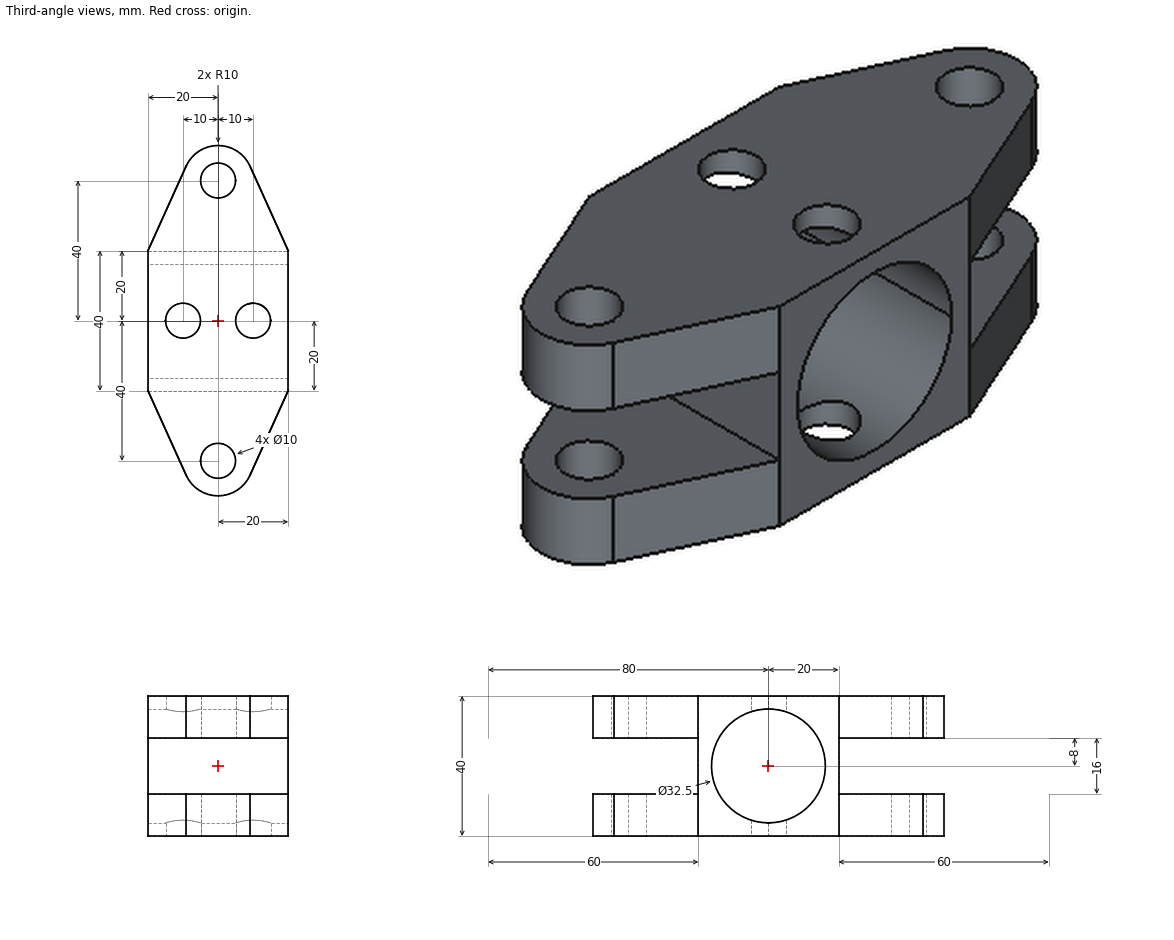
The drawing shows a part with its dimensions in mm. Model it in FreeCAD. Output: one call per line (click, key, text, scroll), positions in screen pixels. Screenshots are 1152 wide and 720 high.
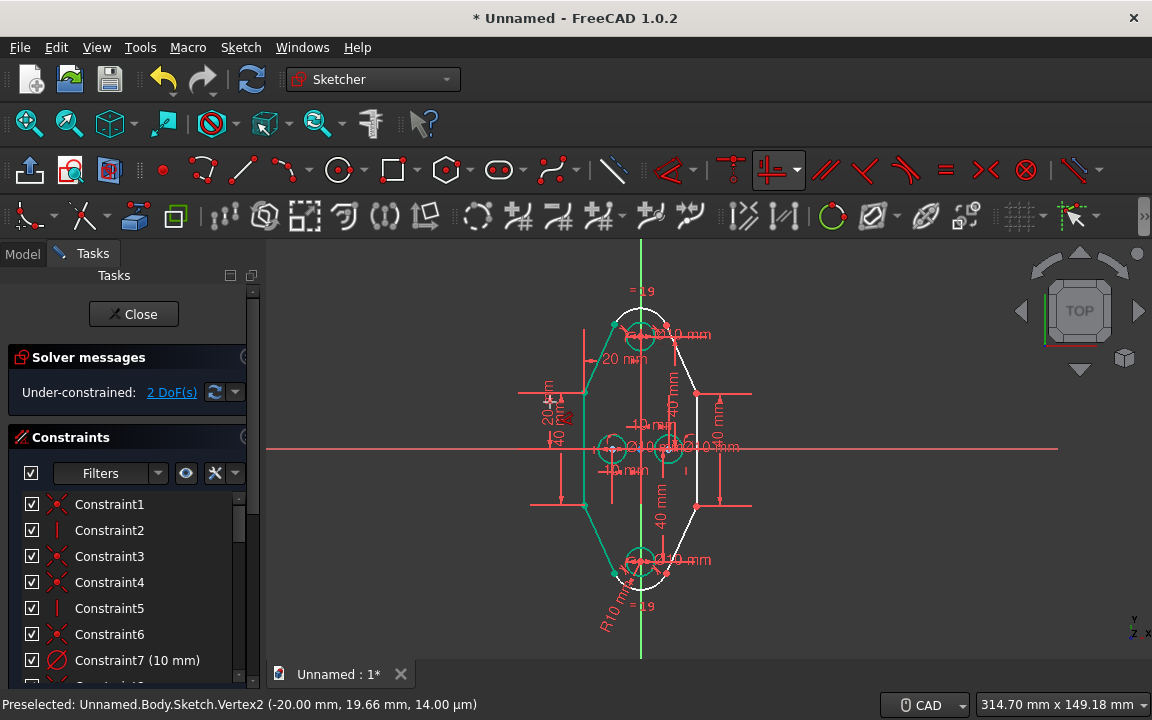
click(697, 506)
click(689, 564)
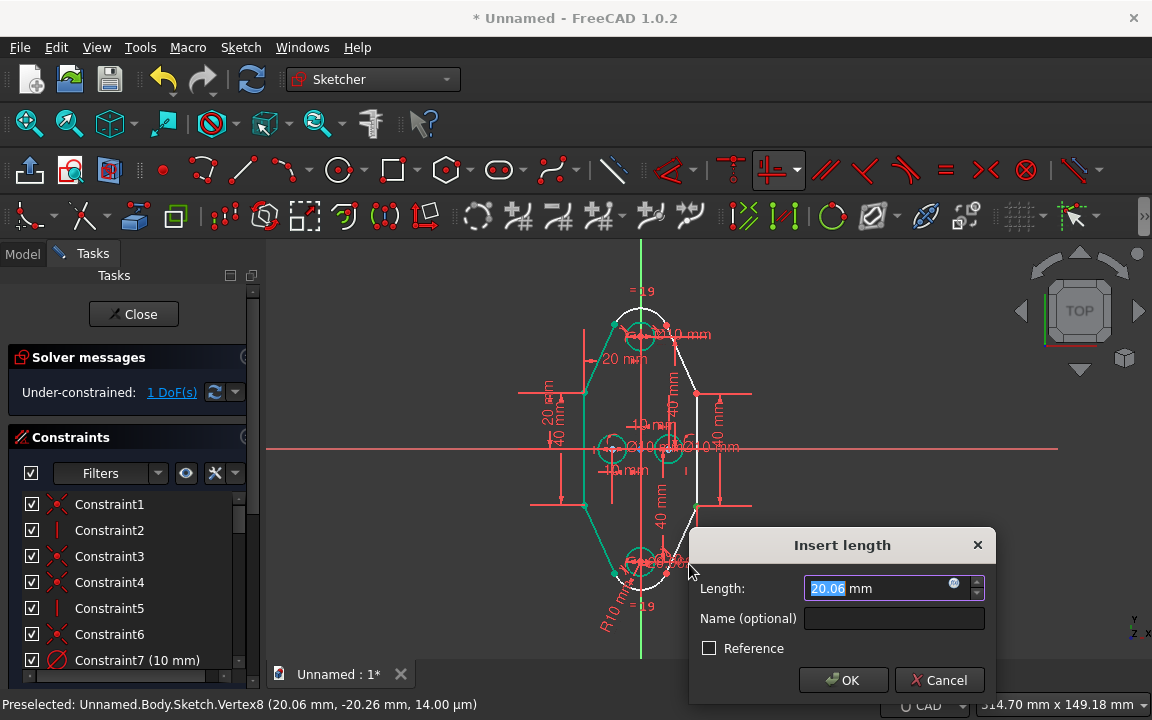
text(20)
key(Return)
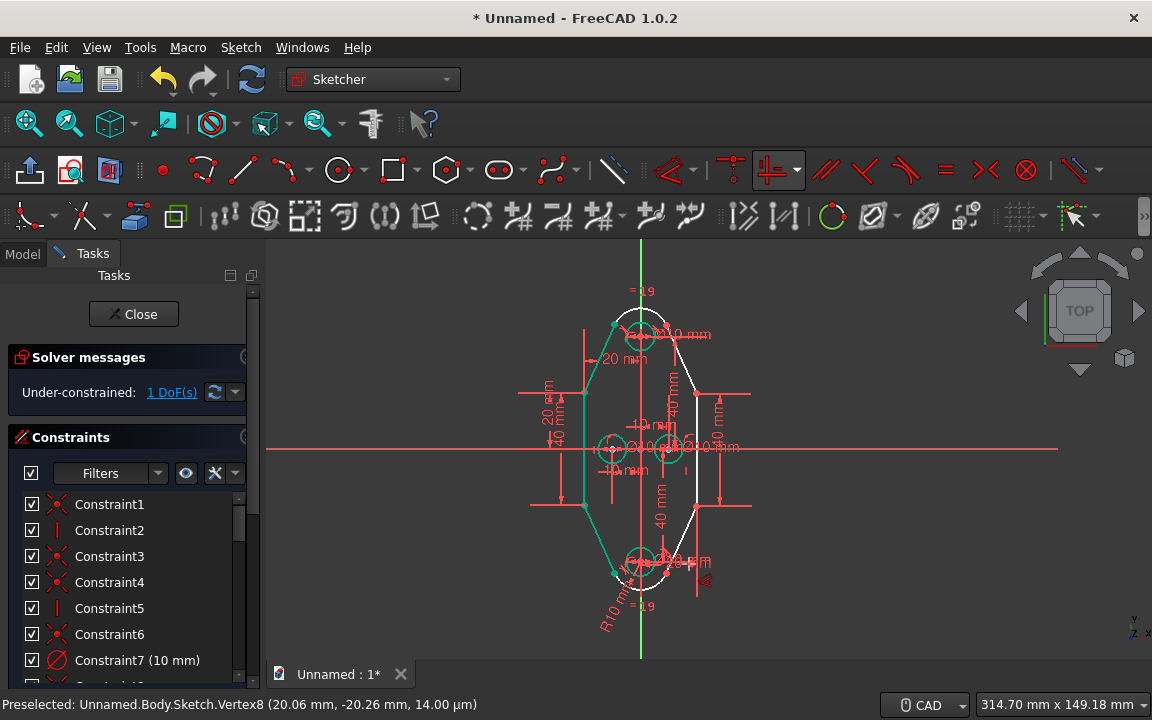
click(697, 506)
click(731, 478)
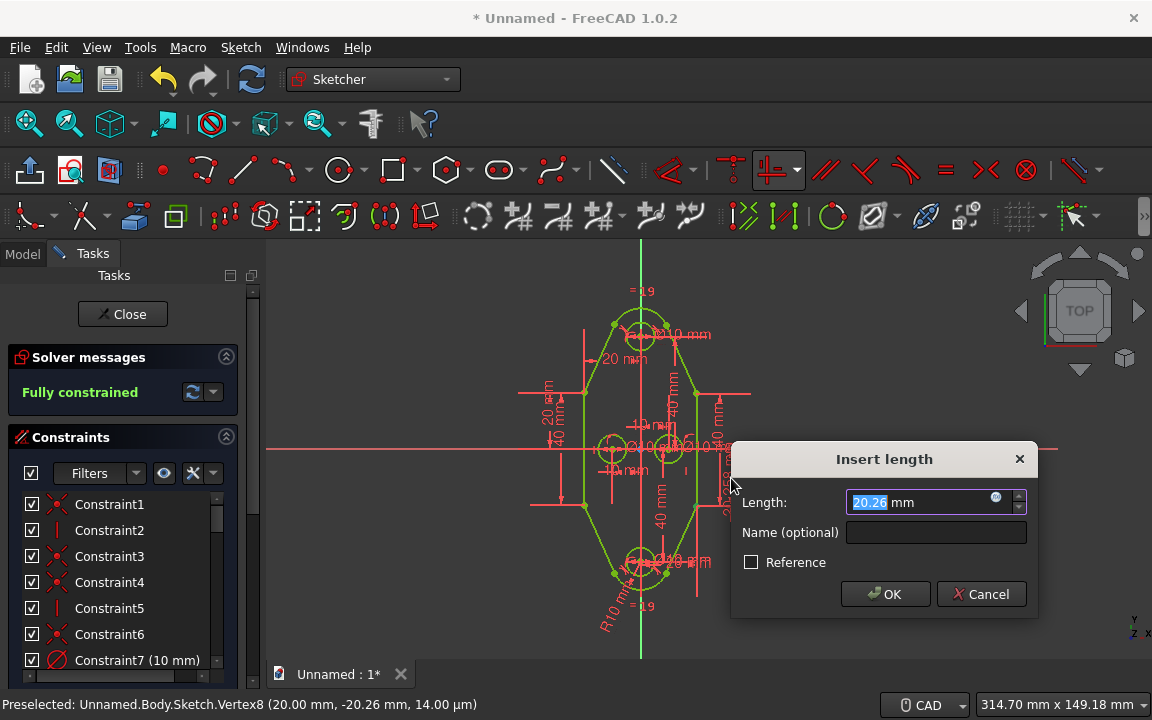
text(20)
key(Return)
key(Escape)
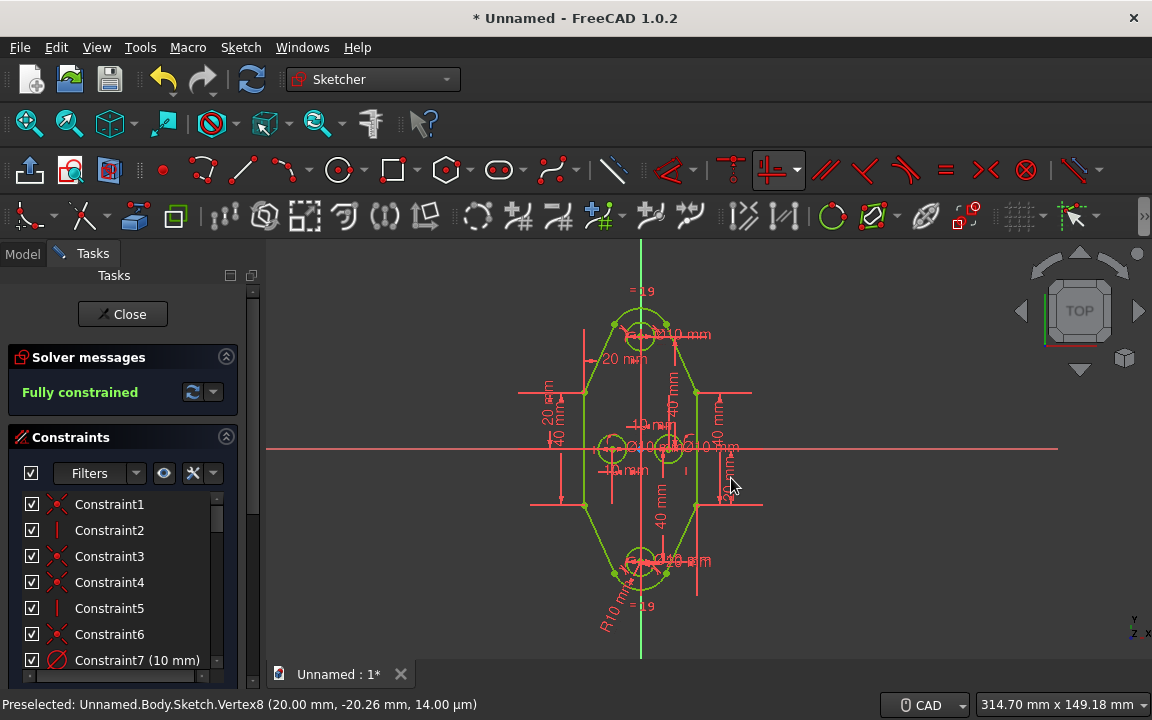
click(123, 314)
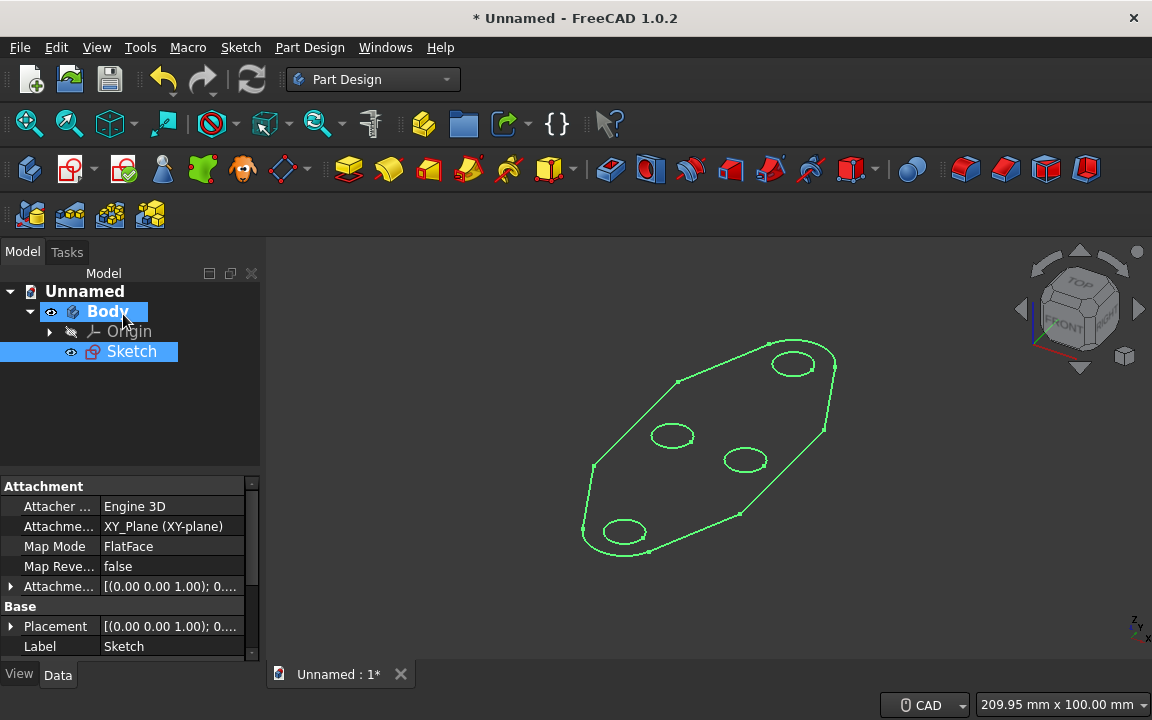
click(350, 170)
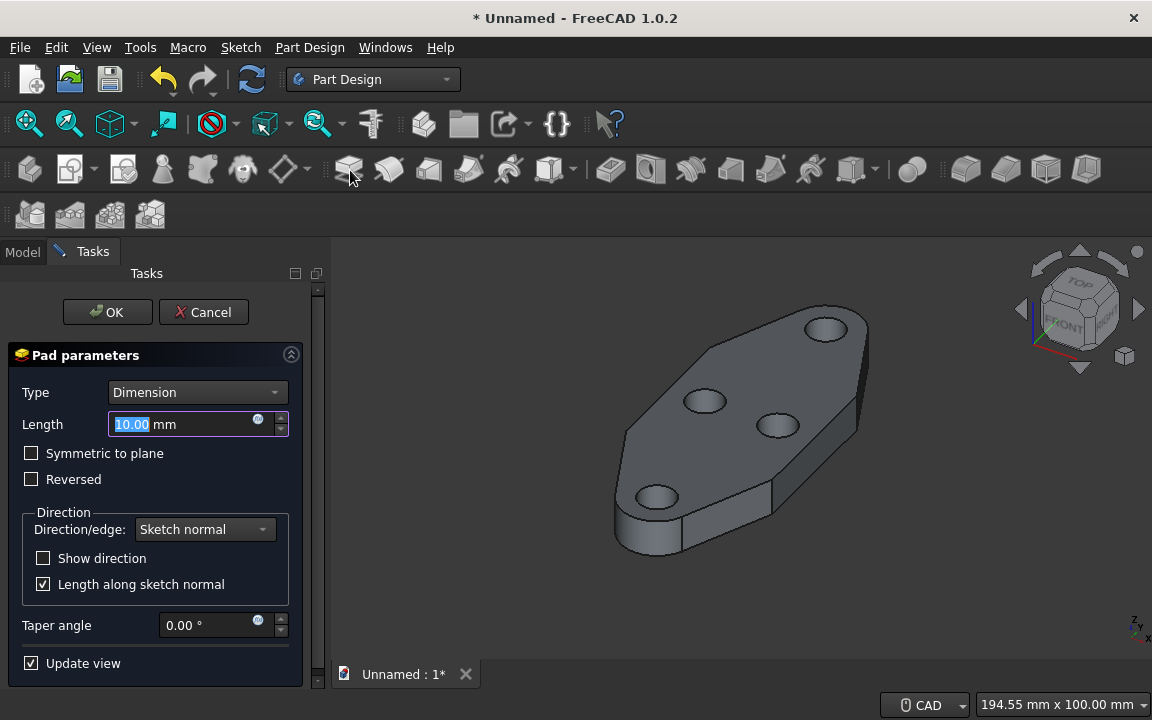
text(40)
key(Tab)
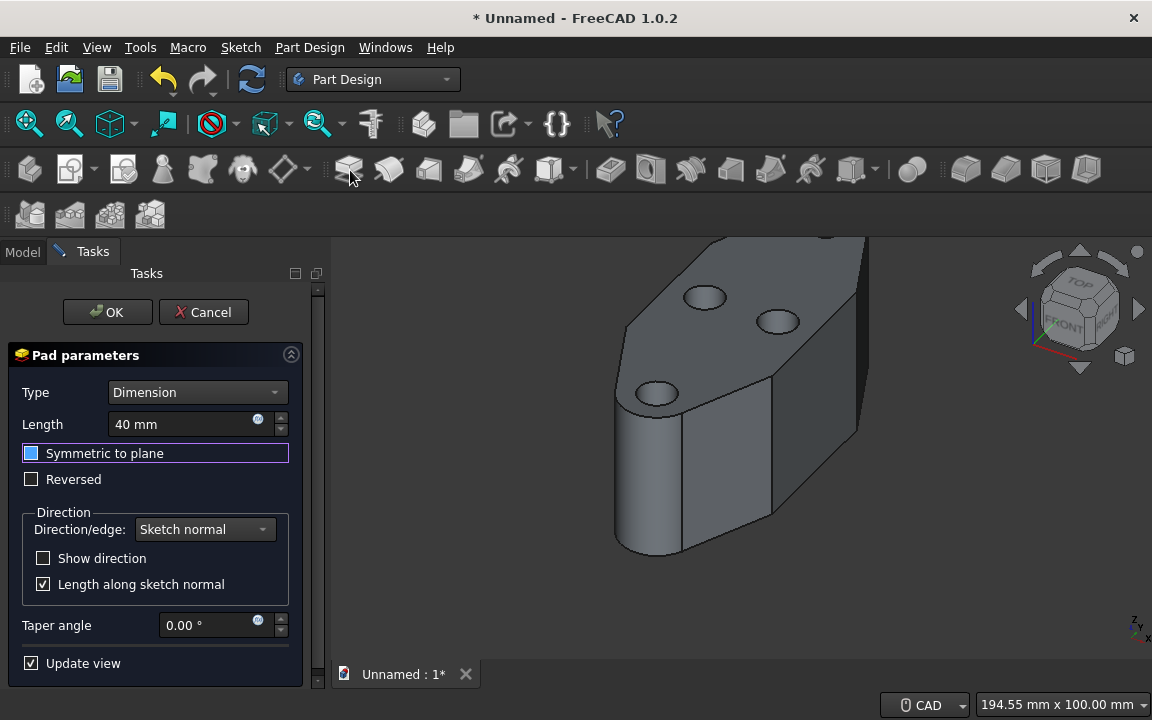
click(30, 453)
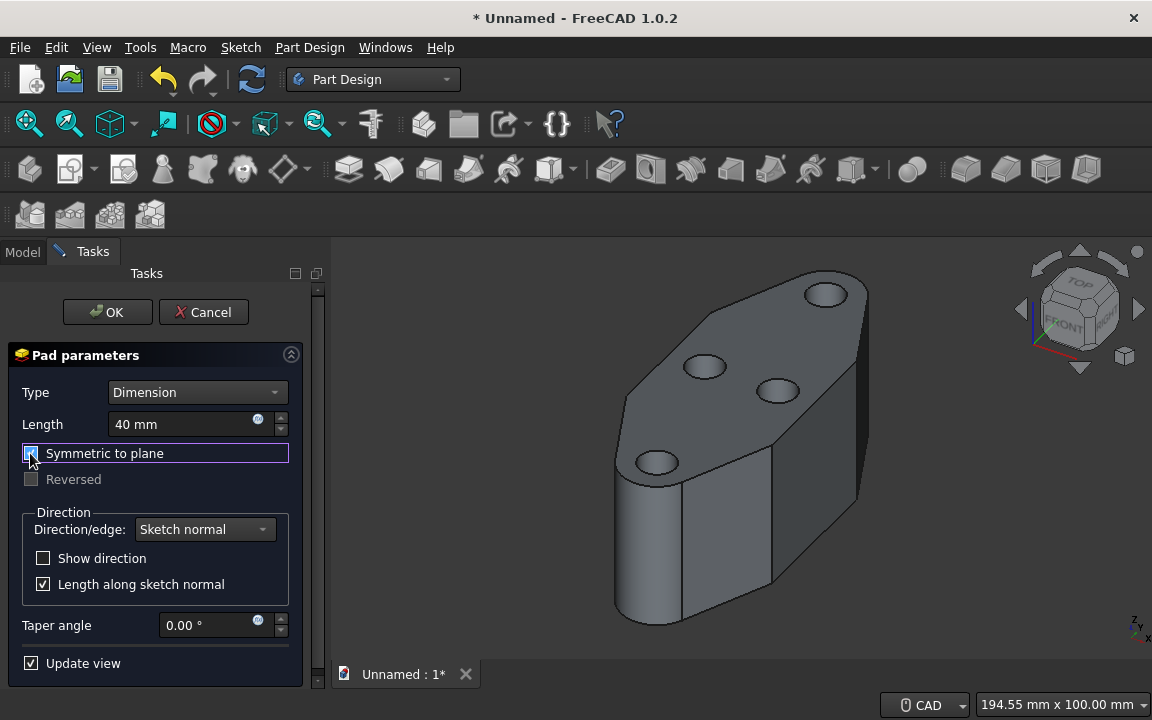
click(108, 312)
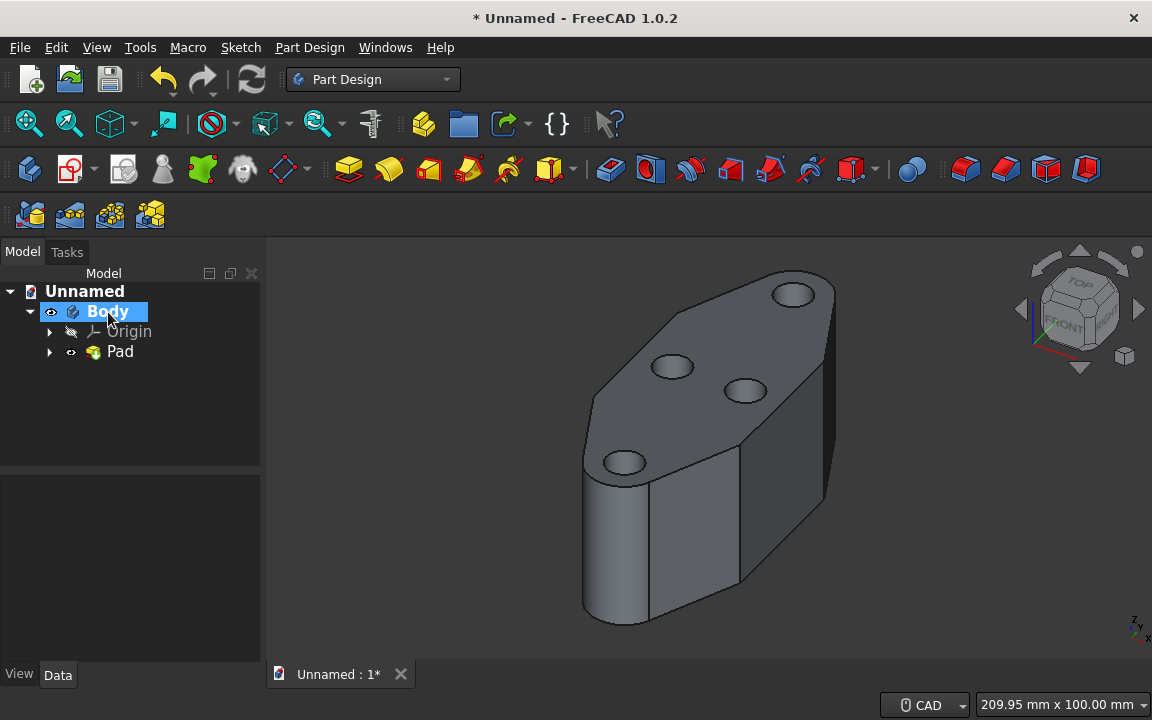
click(70, 170)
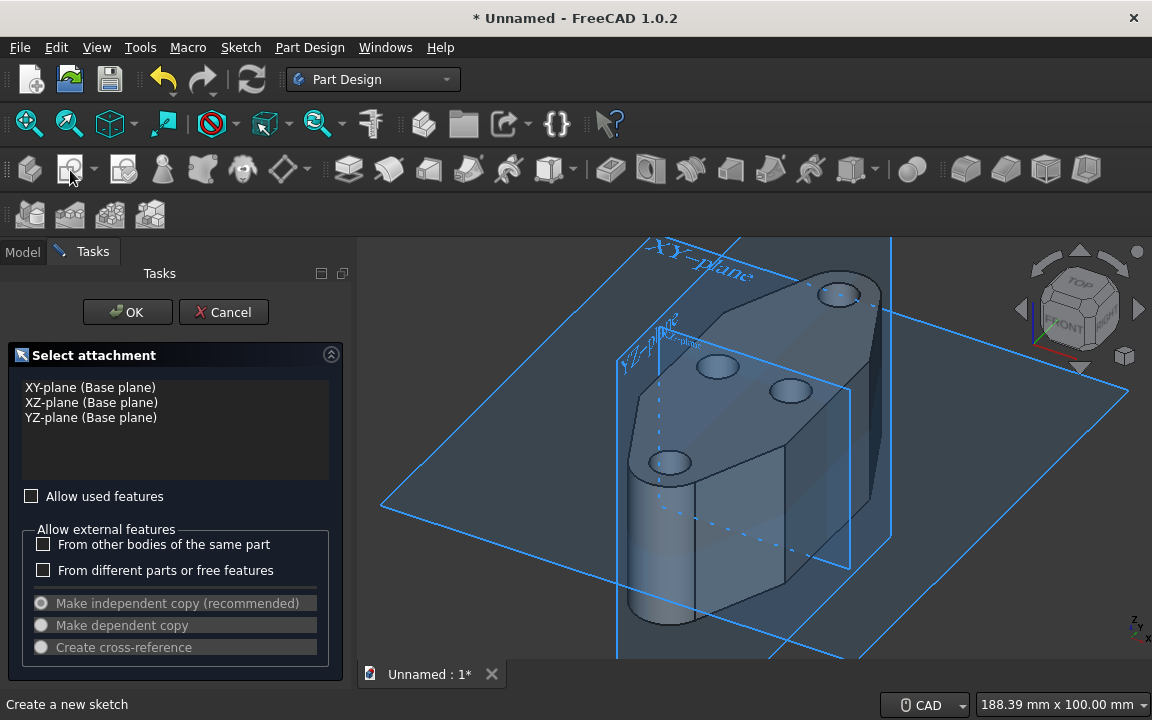
click(82, 418)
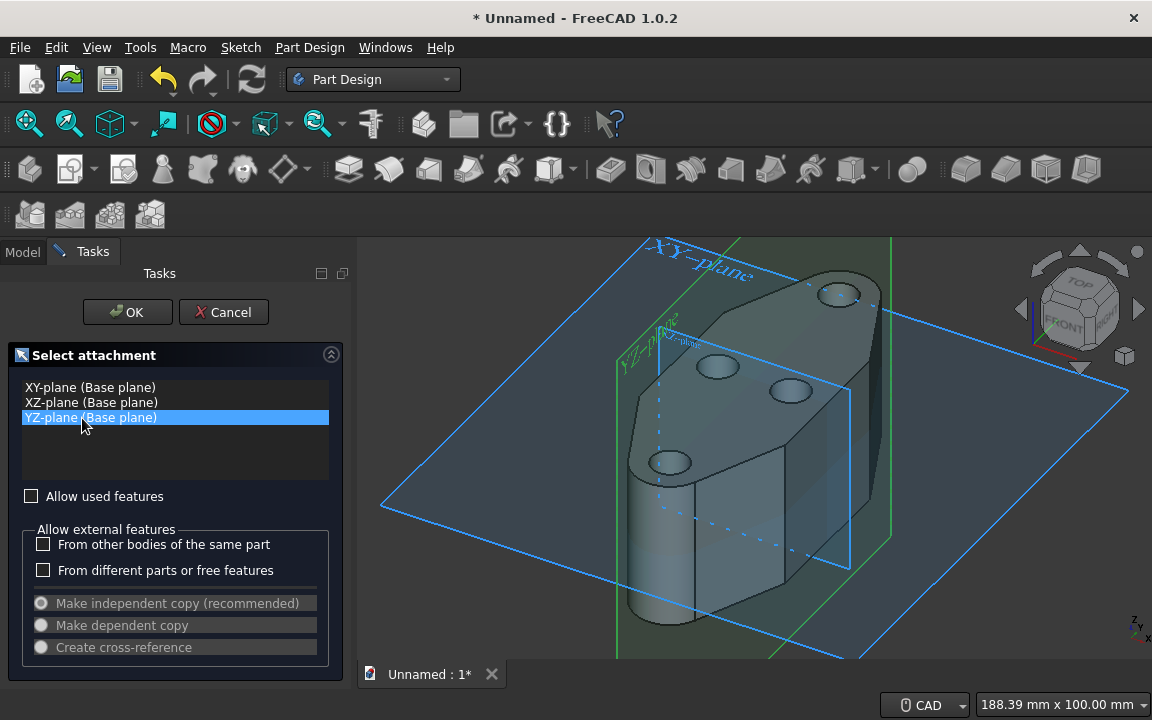
click(128, 312)